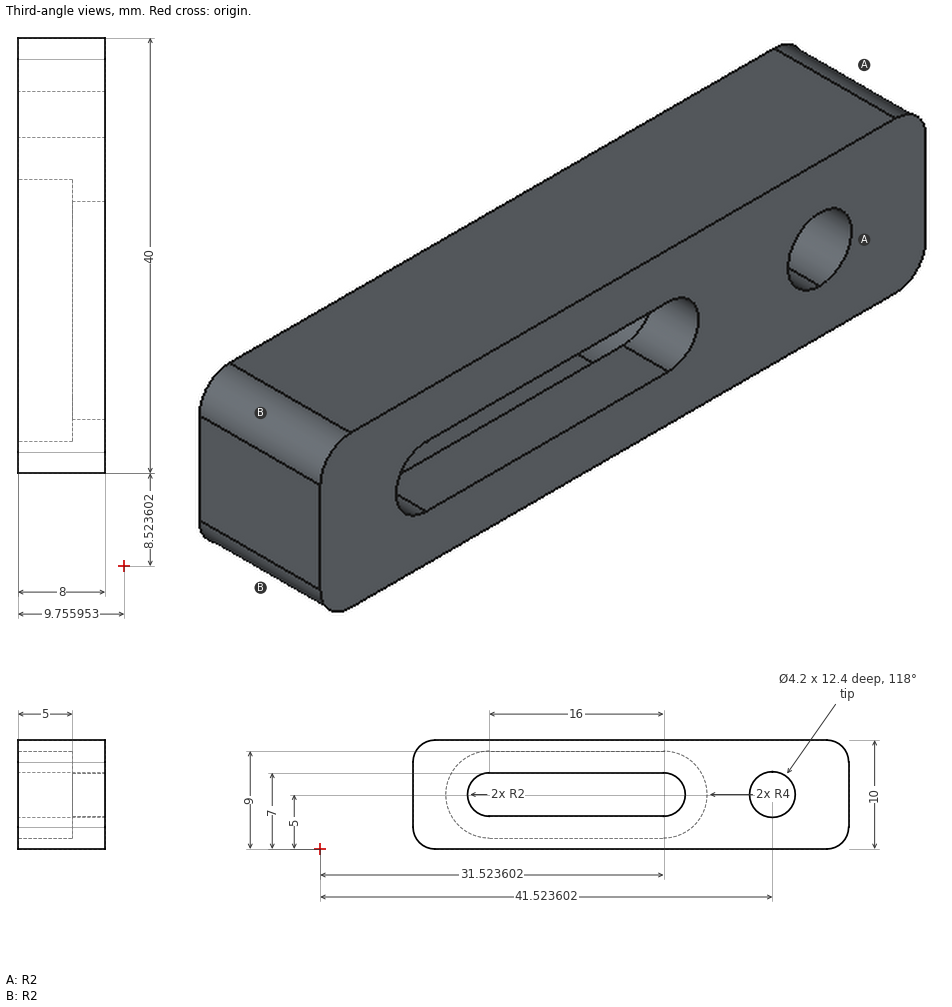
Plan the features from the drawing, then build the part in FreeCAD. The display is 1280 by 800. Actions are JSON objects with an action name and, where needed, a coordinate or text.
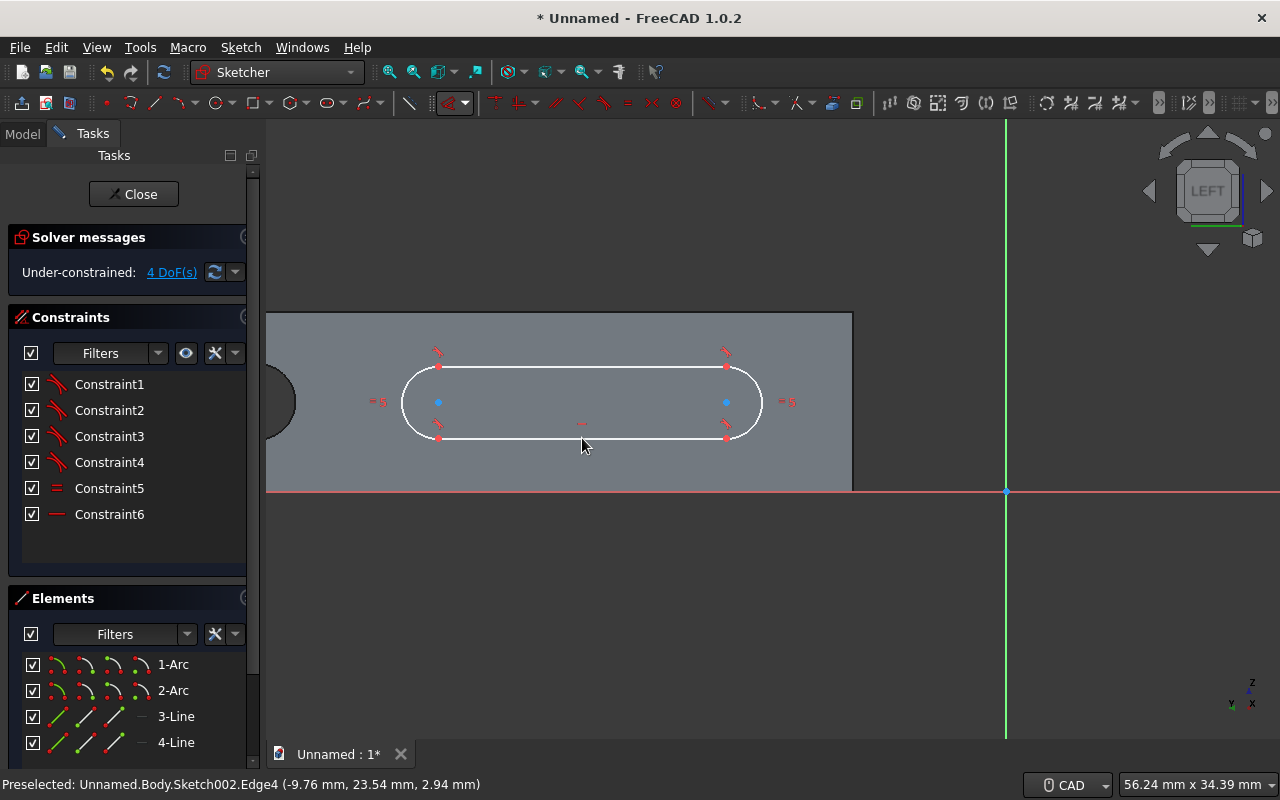
{"action": "key", "text": "d"}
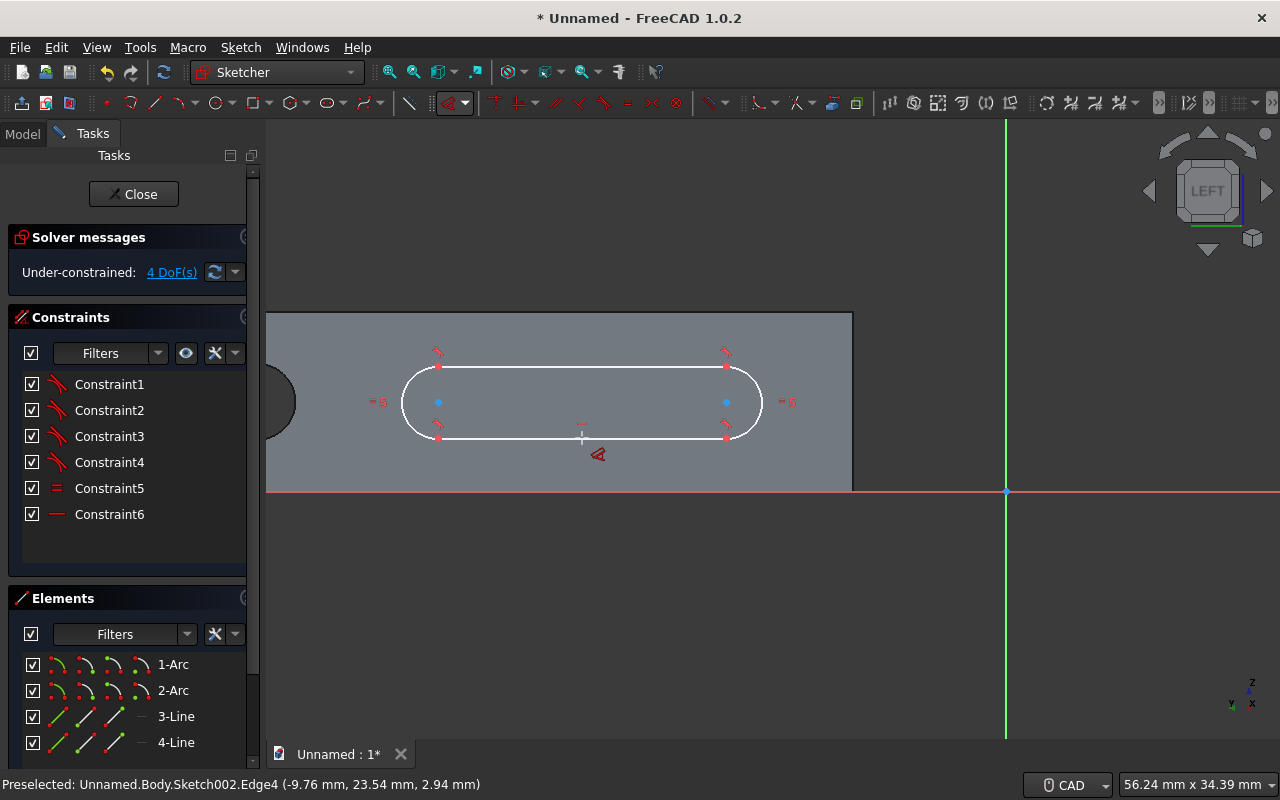
{"action": "left_click", "coordinate": [409, 382]}
{"action": "left_click", "coordinate": [383, 363]}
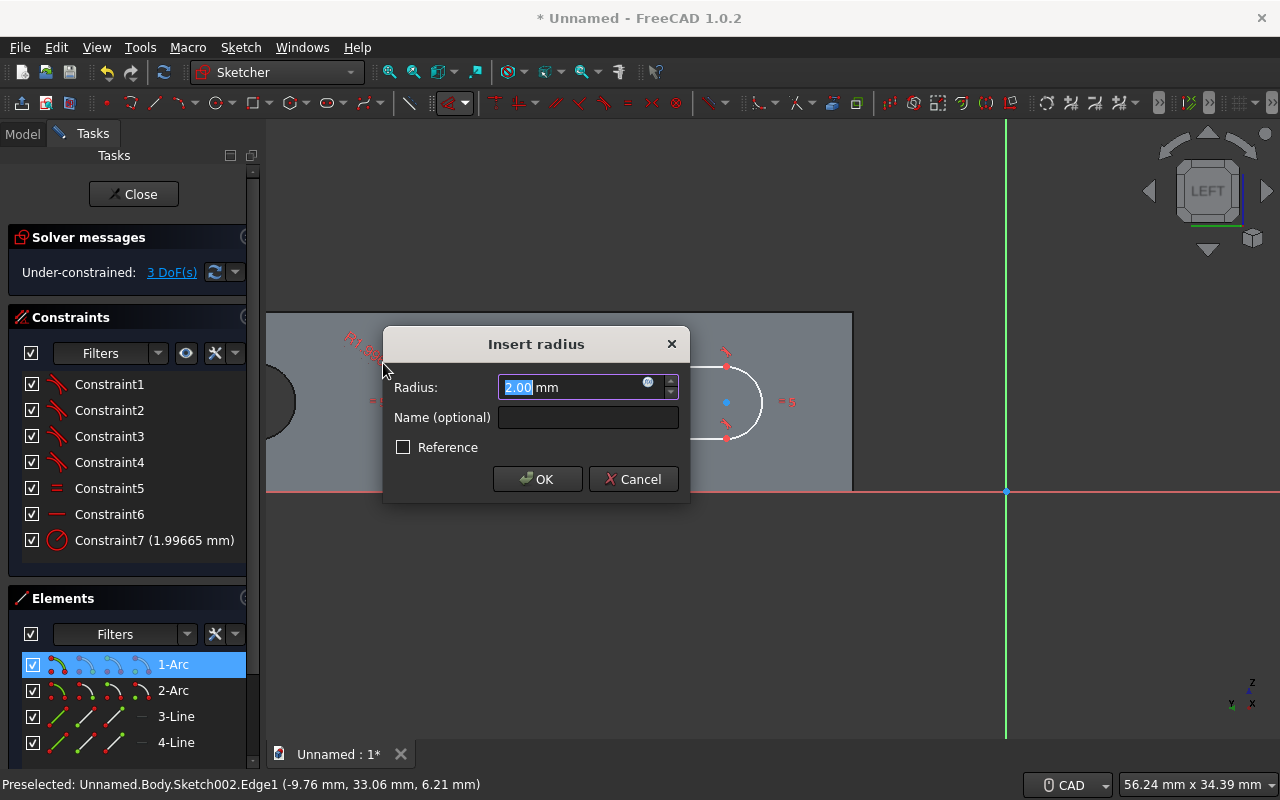
{"action": "type", "text": "2"}
{"action": "key", "text": "Return"}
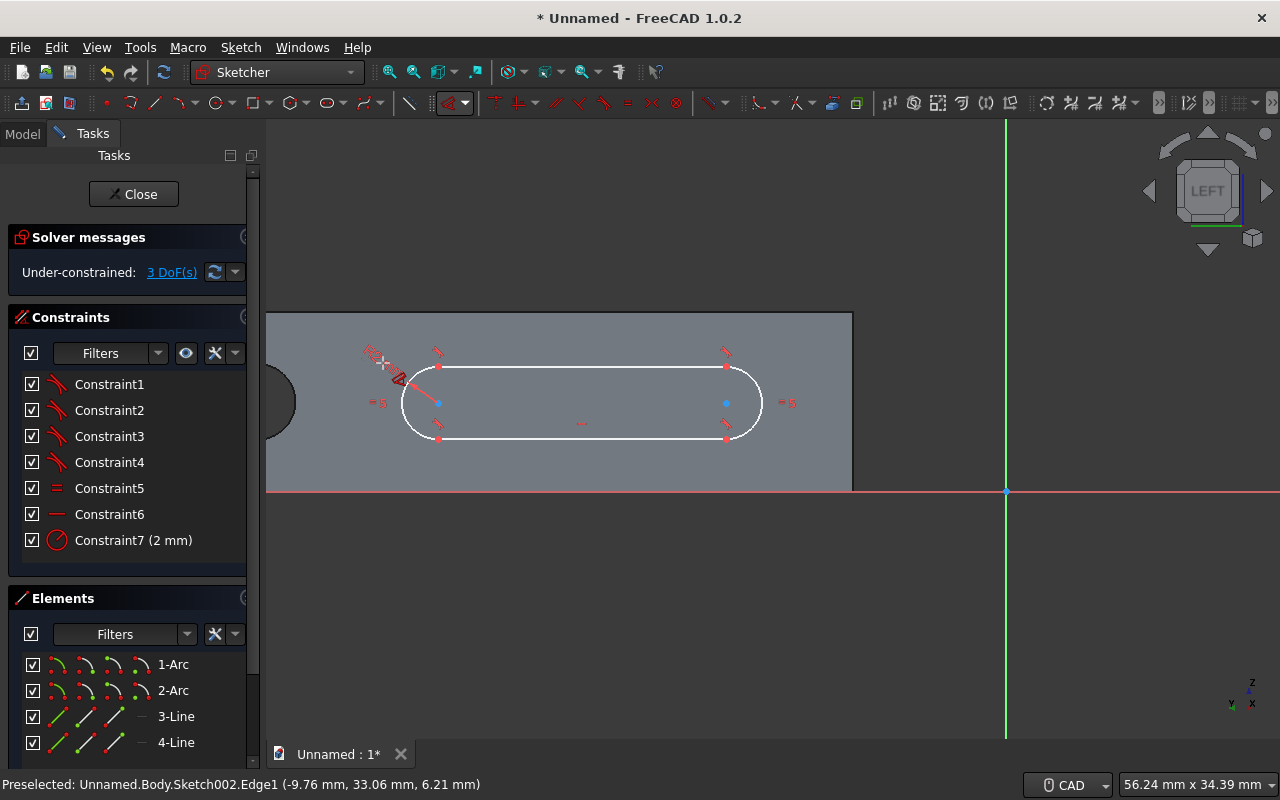
{"action": "left_click", "coordinate": [524, 367]}
{"action": "left_click", "coordinate": [582, 333]}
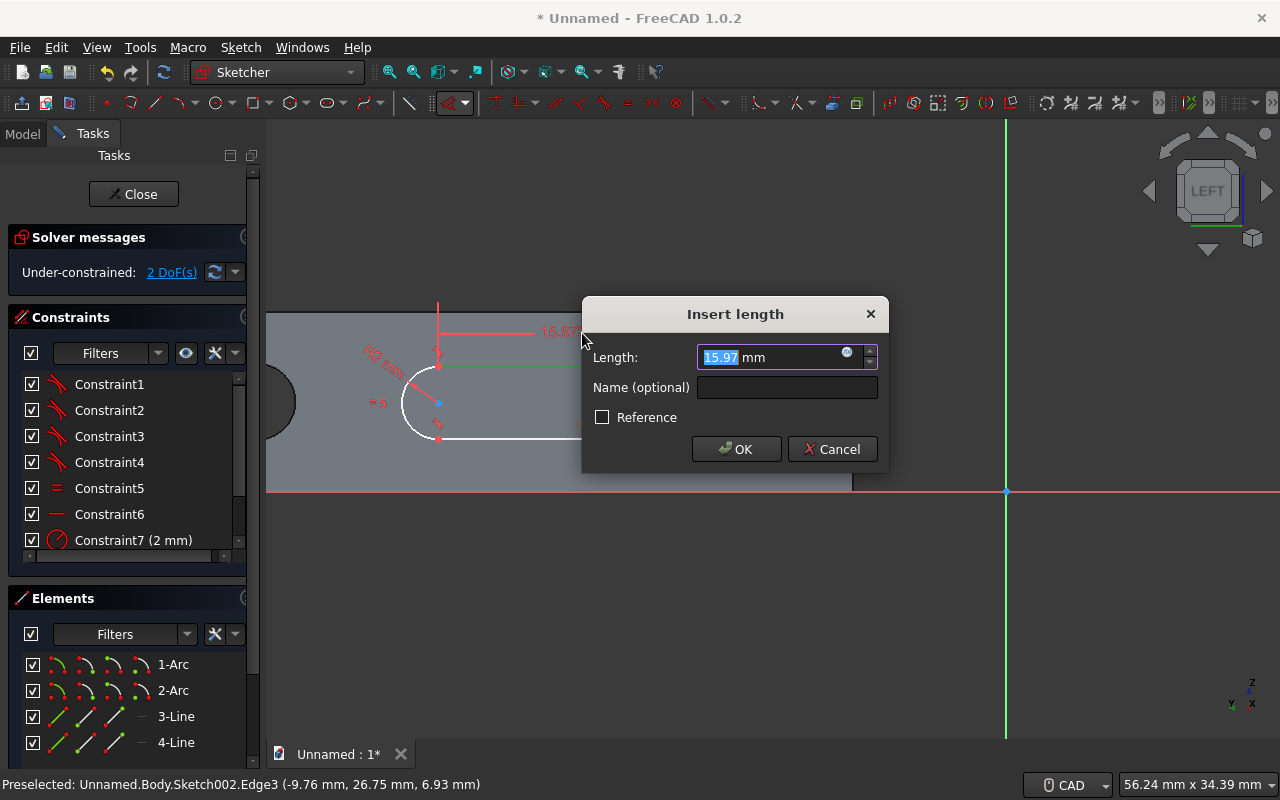
{"action": "type", "text": "16"}
{"action": "key", "text": "Return"}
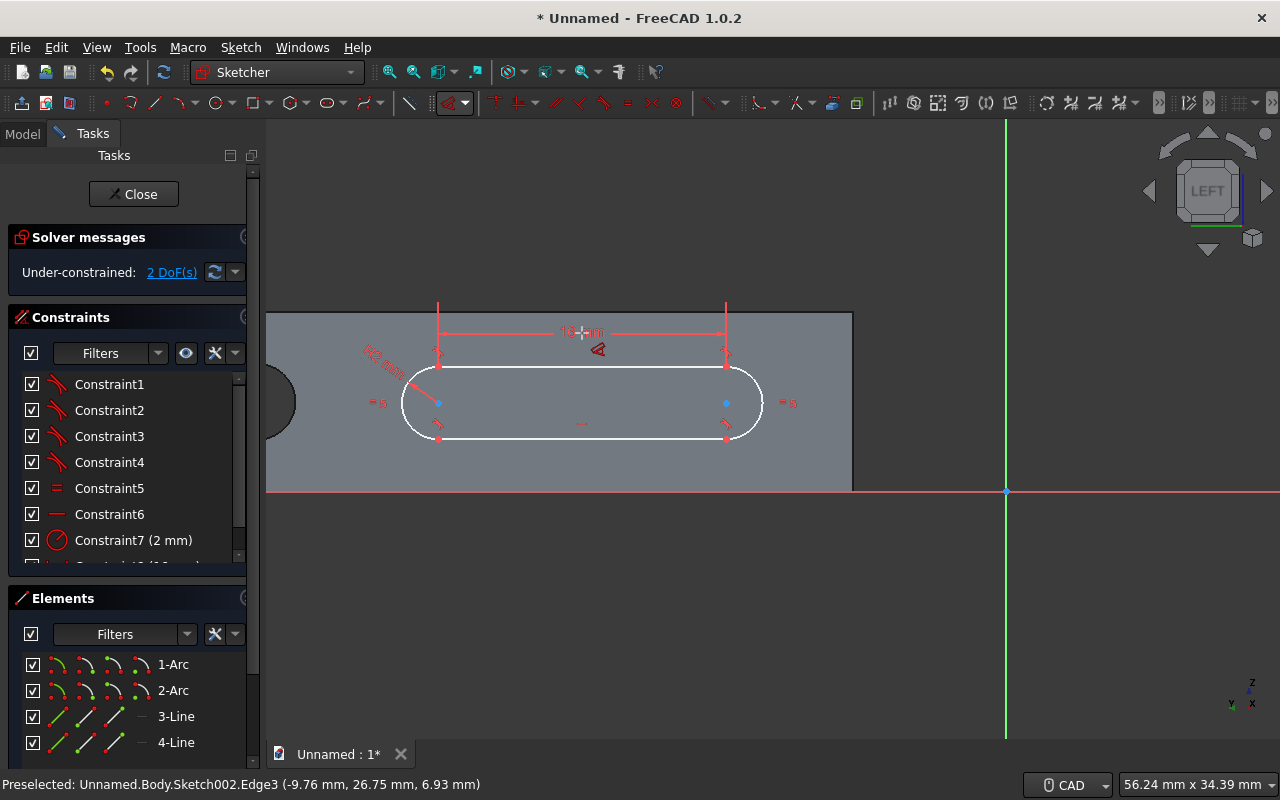
{"action": "left_click", "coordinate": [438, 367]}
{"action": "left_click", "coordinate": [1040, 429]}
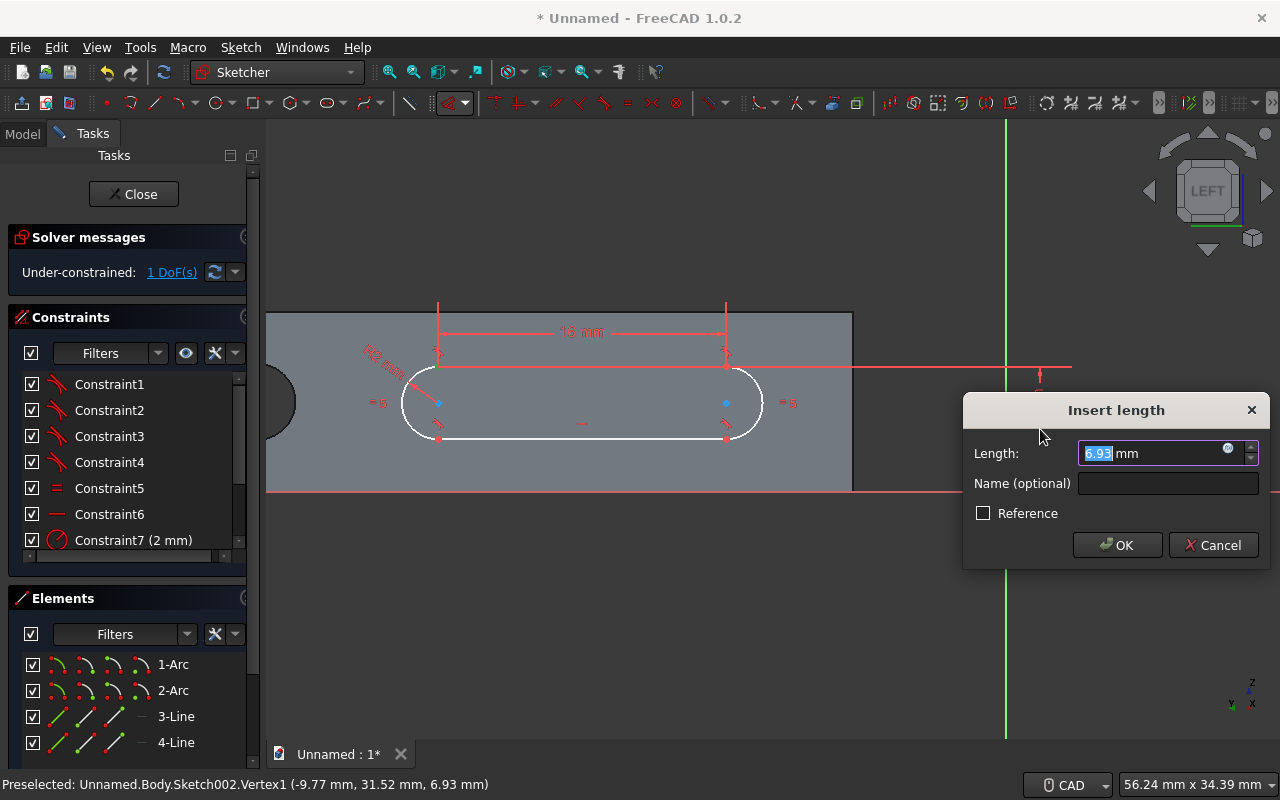
{"action": "type", "text": "7"}
{"action": "key", "text": "Return"}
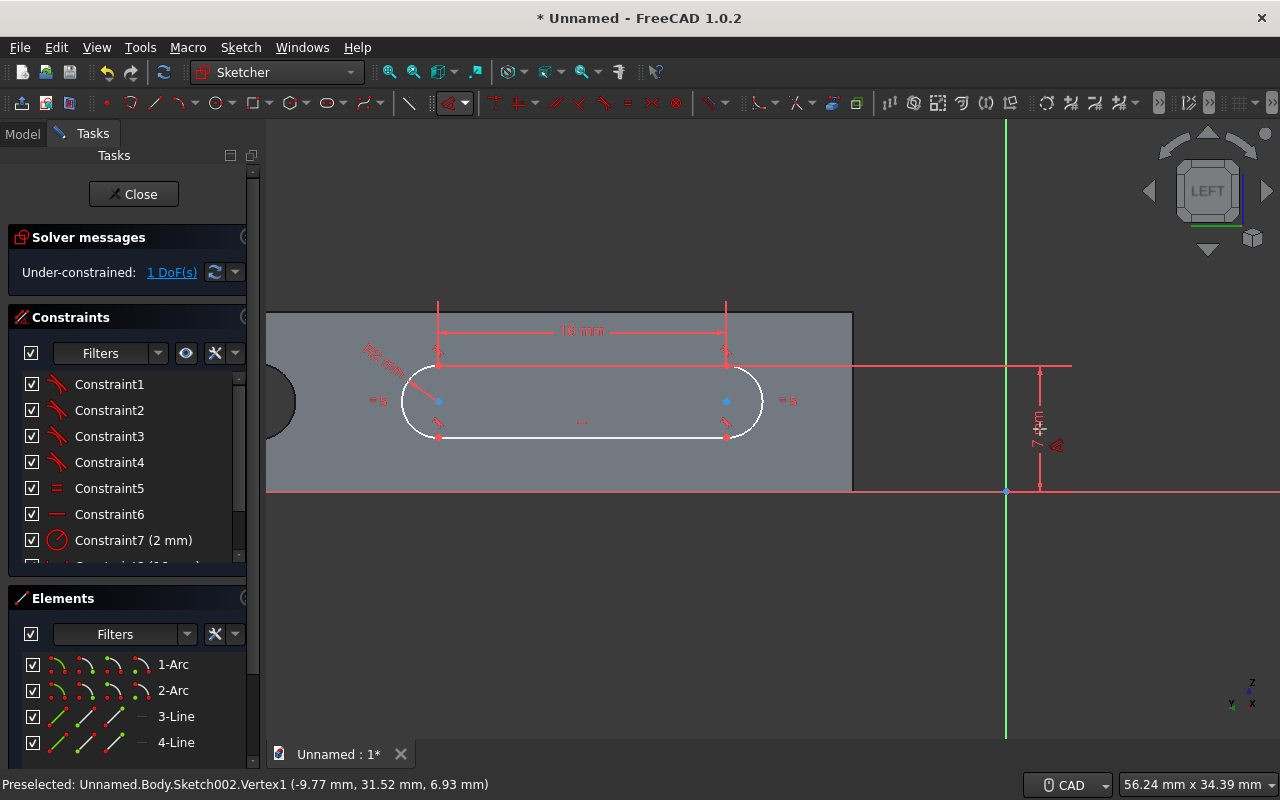
{"action": "left_click", "coordinate": [438, 366]}
{"action": "left_click", "coordinate": [722, 526]}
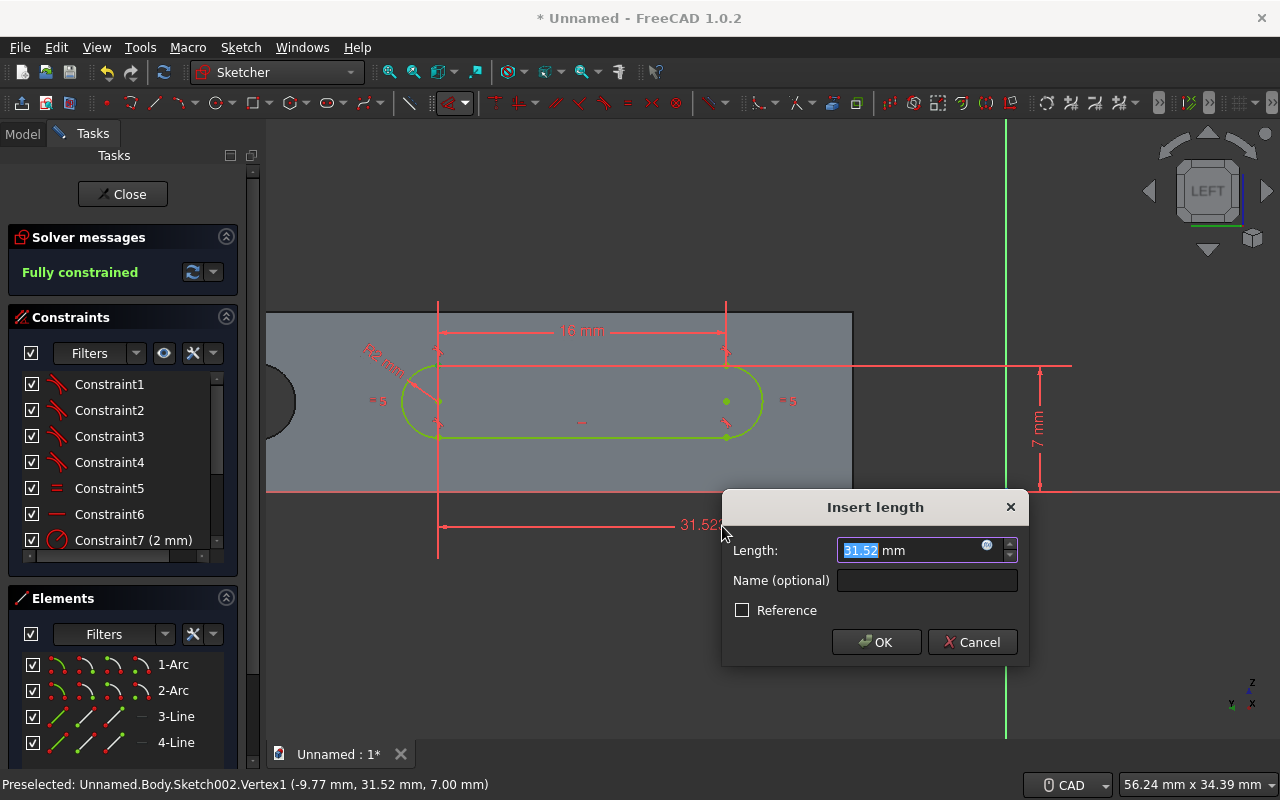
{"action": "type", "text": "31.523602"}
{"action": "key", "text": "Return"}
{"action": "key", "text": "Escape"}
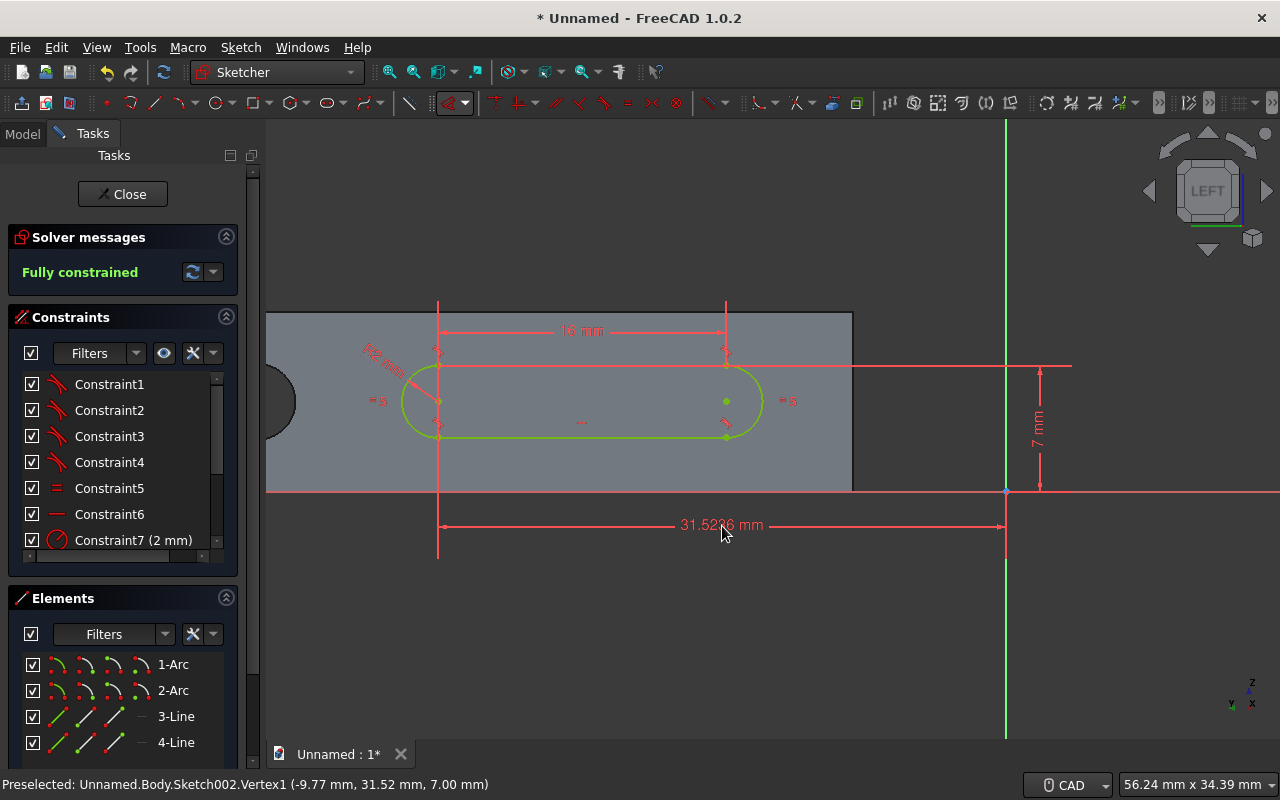
{"action": "left_click", "coordinate": [123, 194]}